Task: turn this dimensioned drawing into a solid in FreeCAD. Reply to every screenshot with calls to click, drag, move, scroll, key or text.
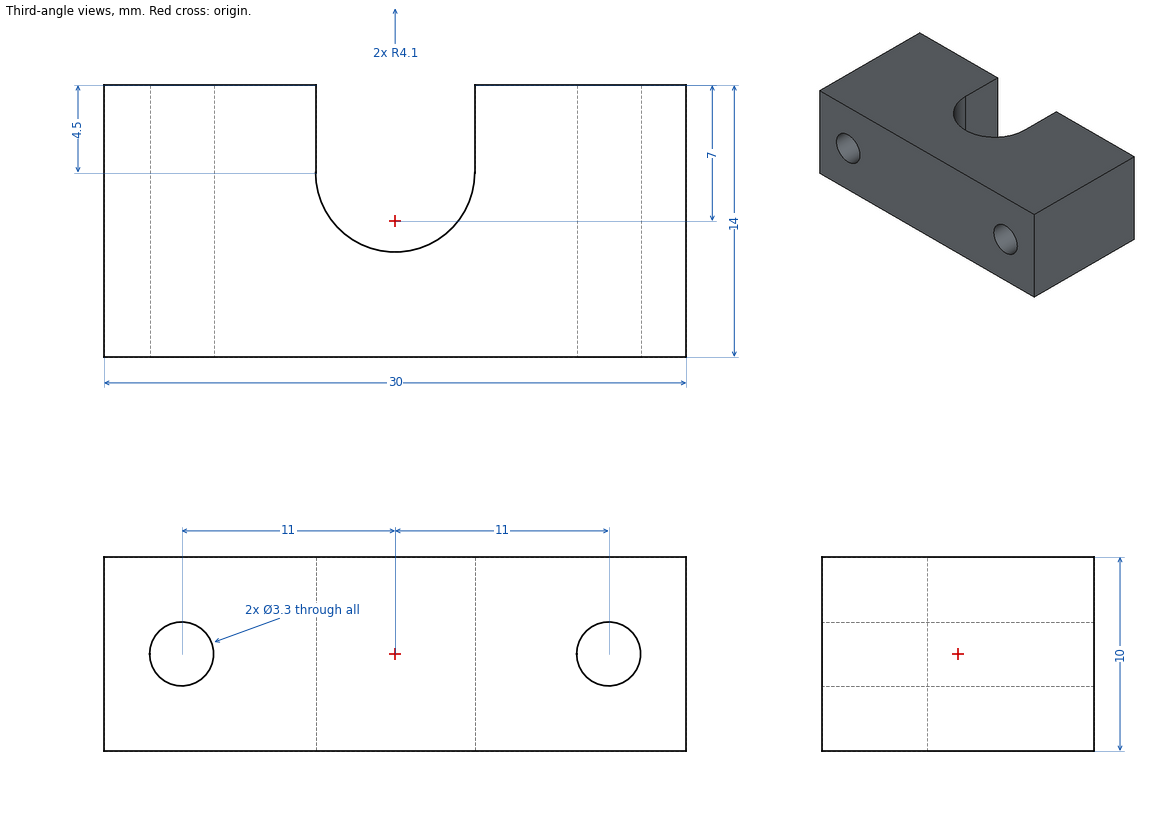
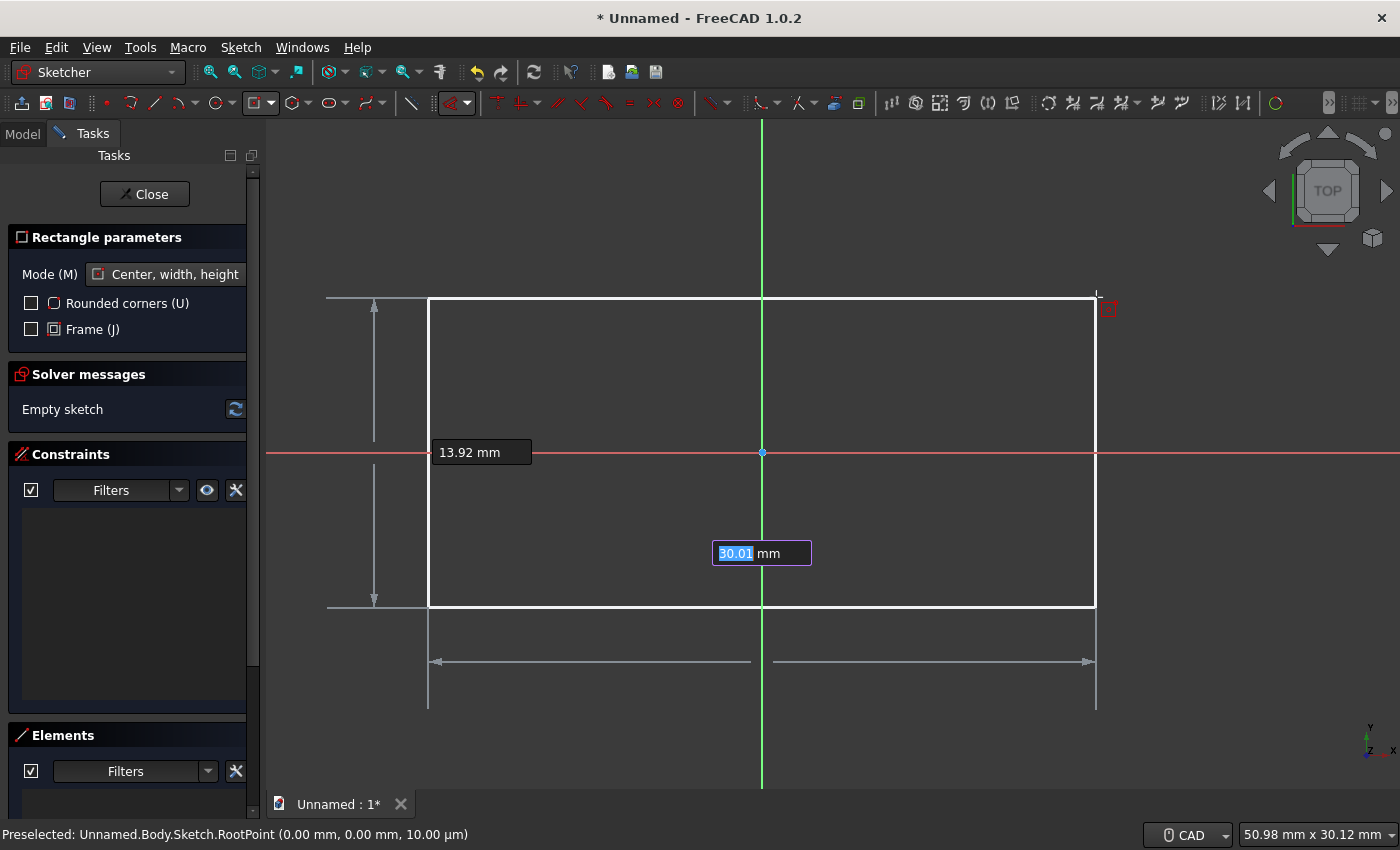
text(30)
key(Tab)
text(14)
key(Return)
key(Escape)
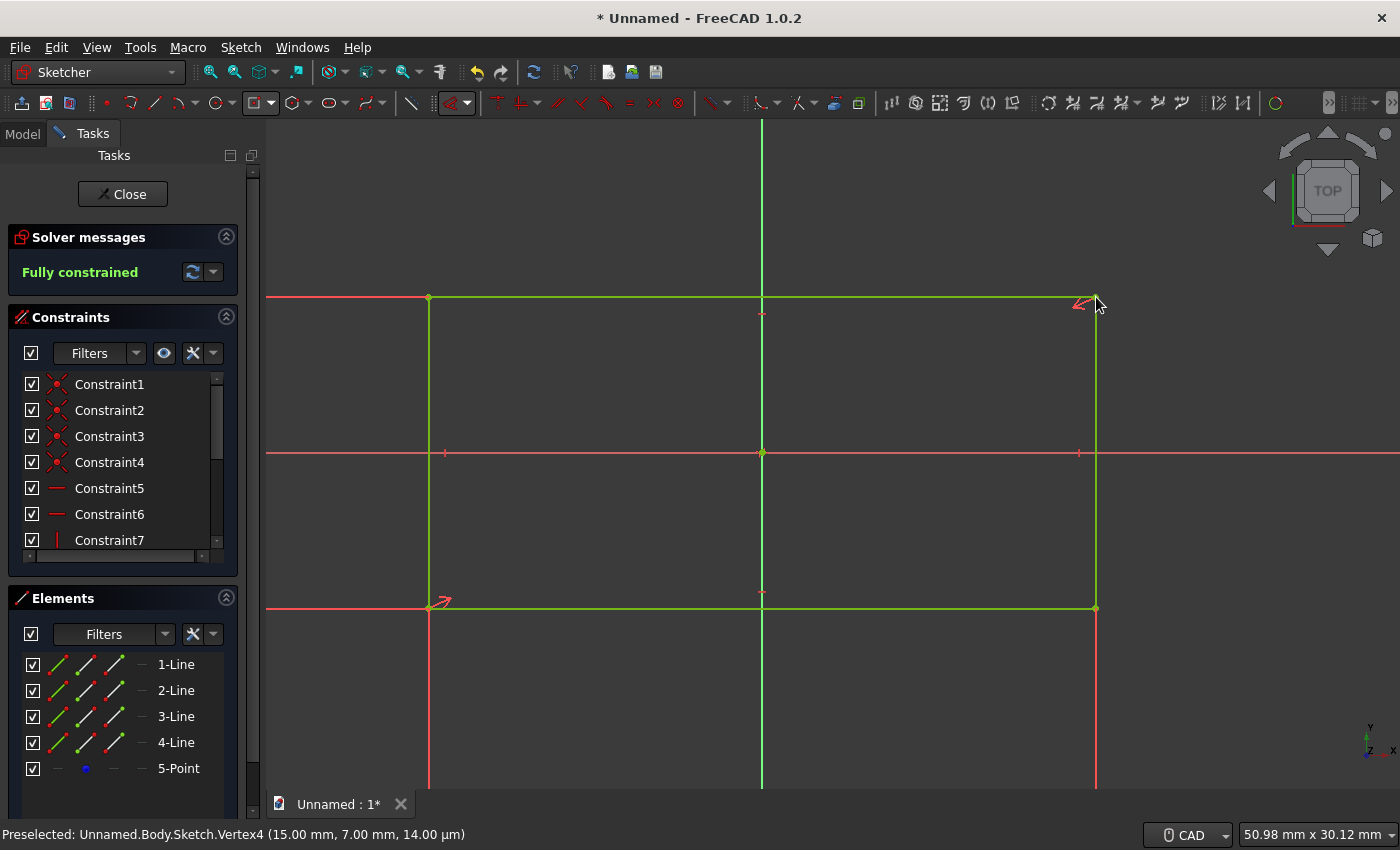
click(123, 194)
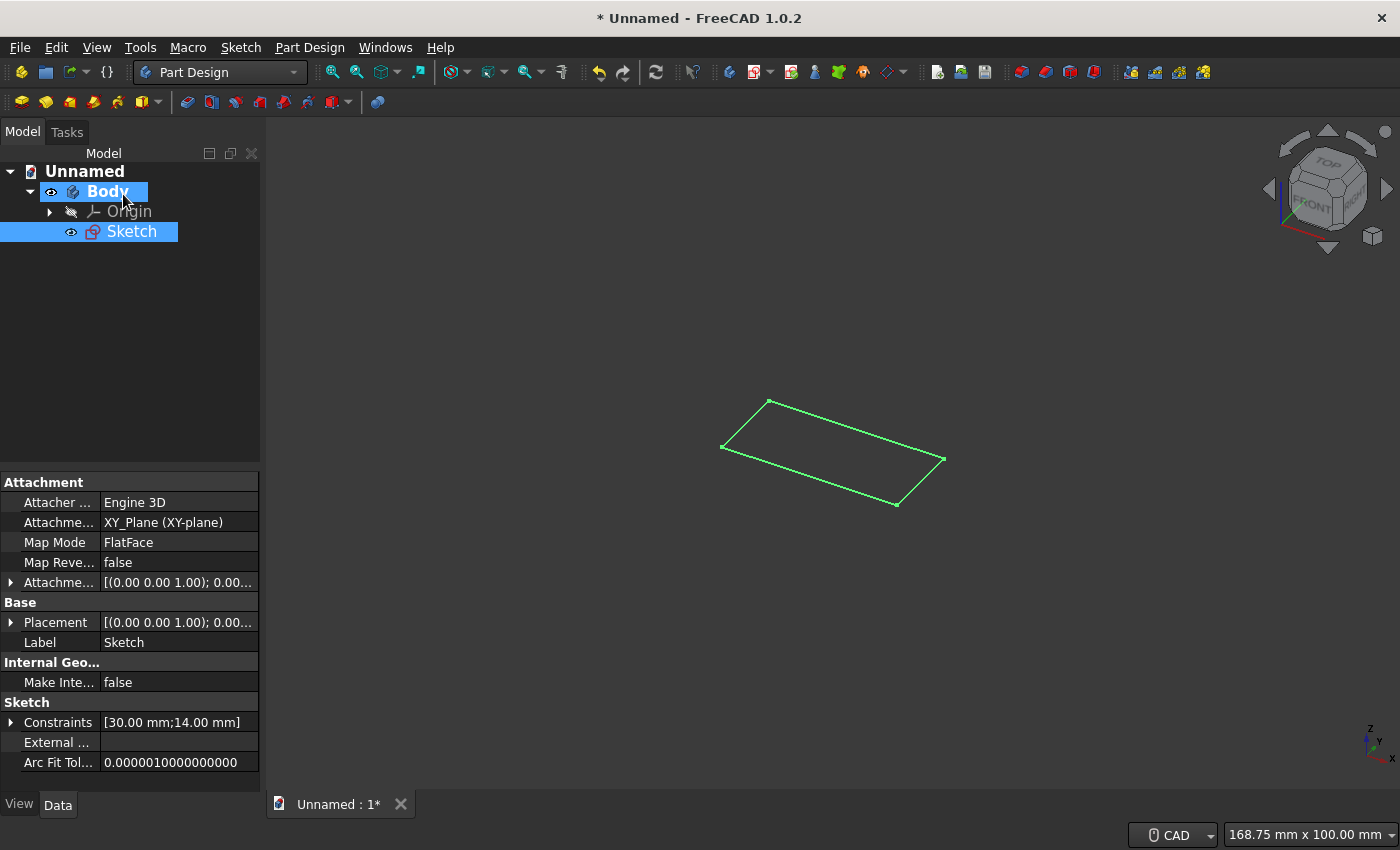
click(22, 102)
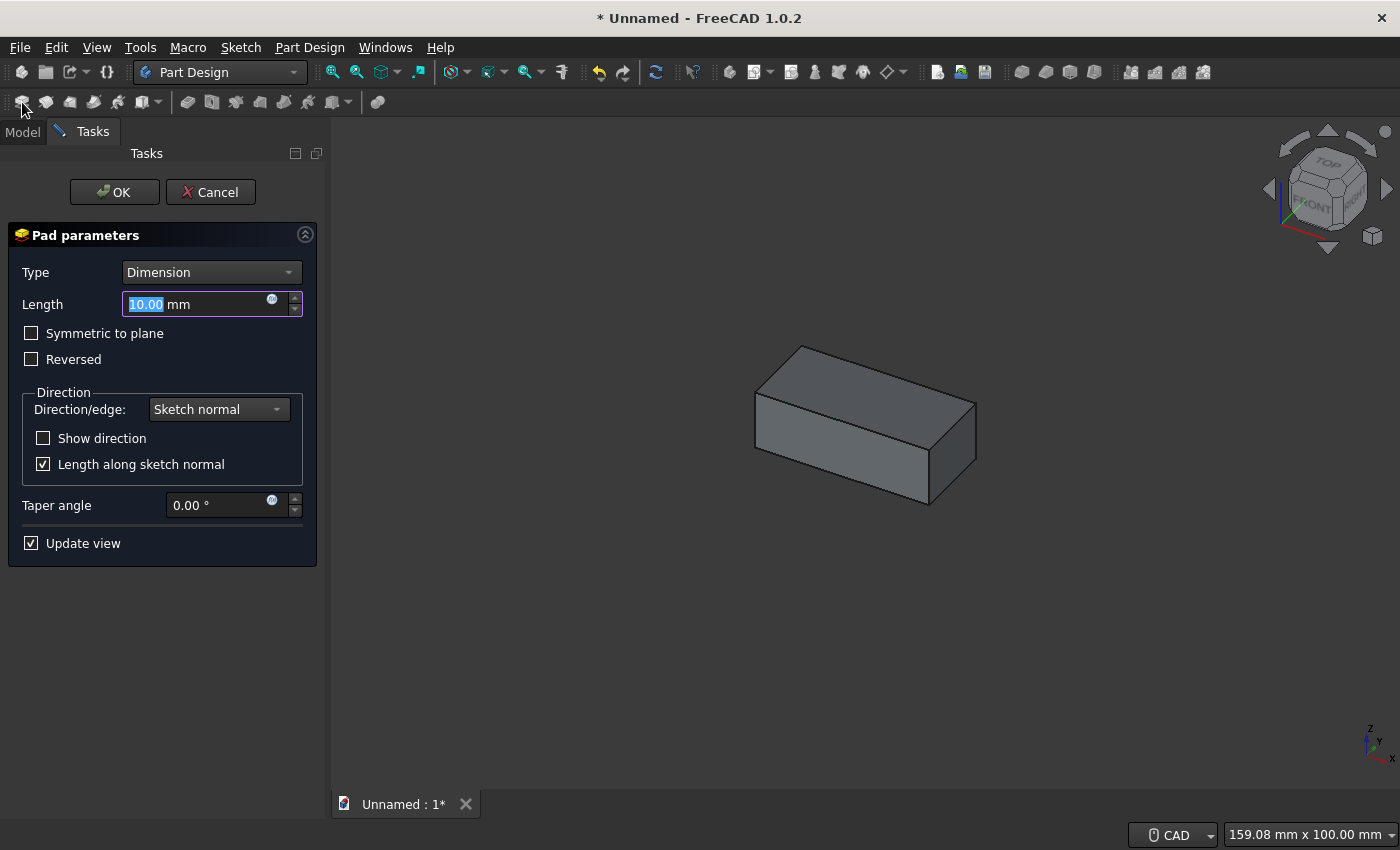
text(10)
key(Tab)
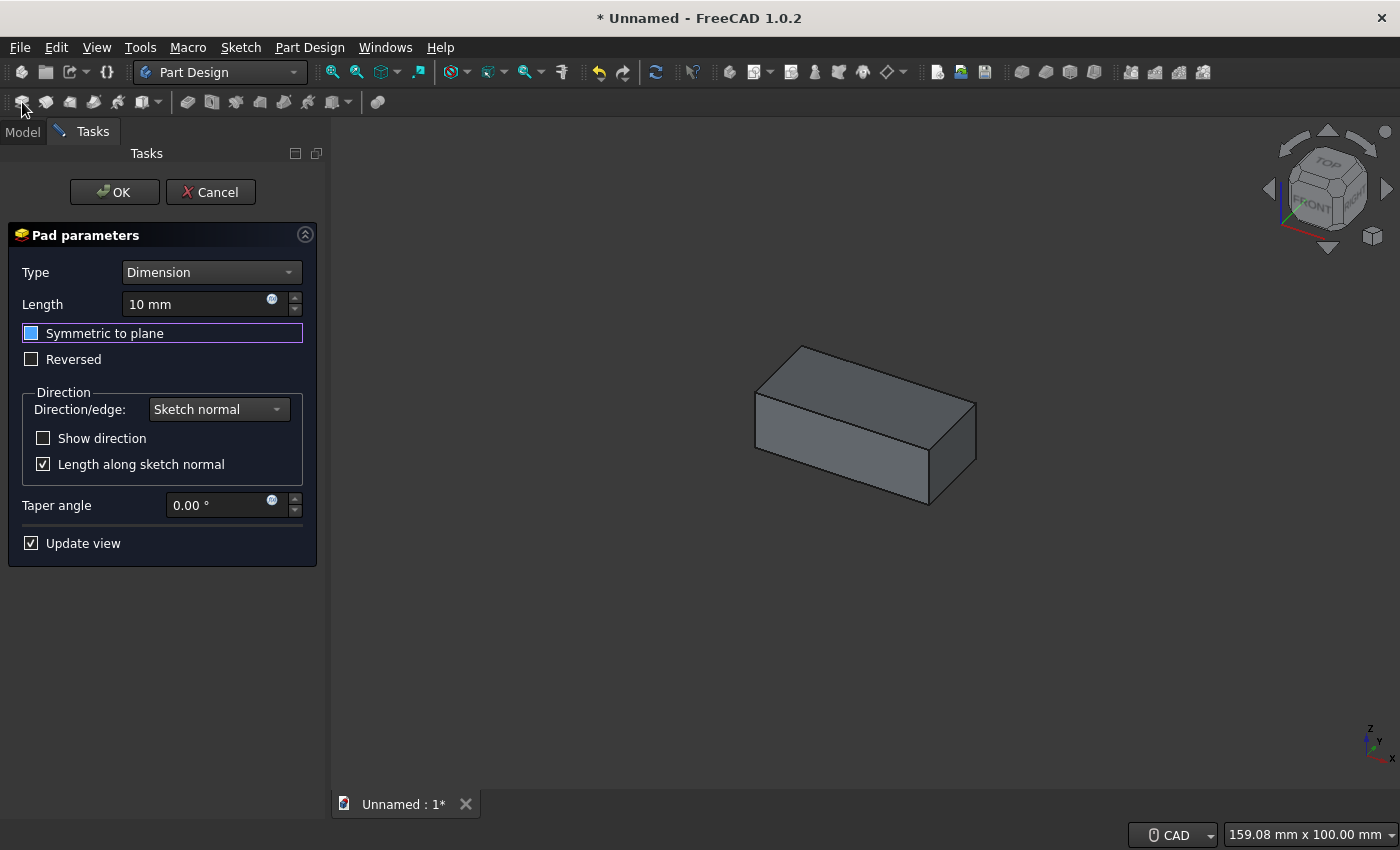
click(30, 333)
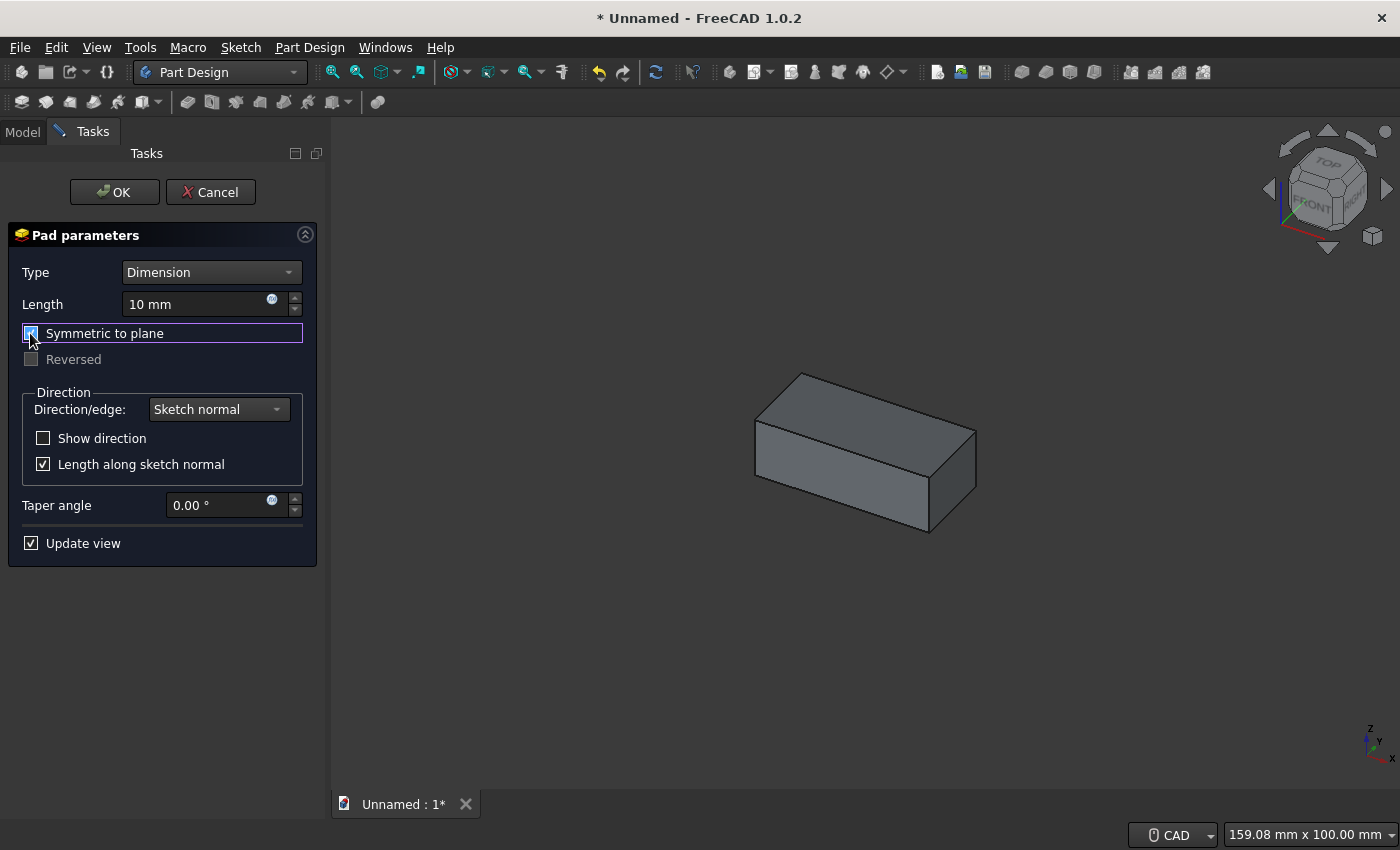
click(115, 192)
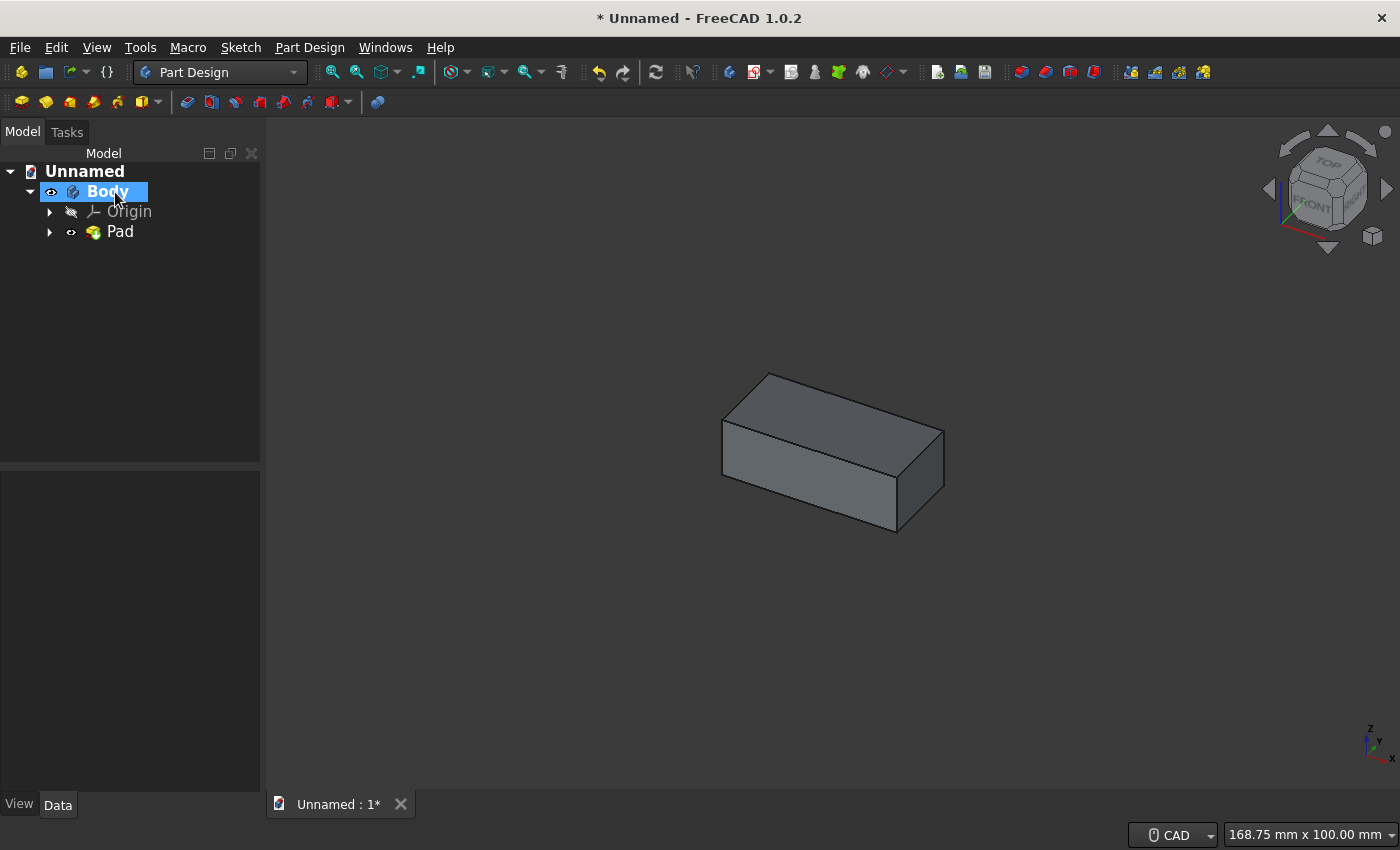
click(334, 72)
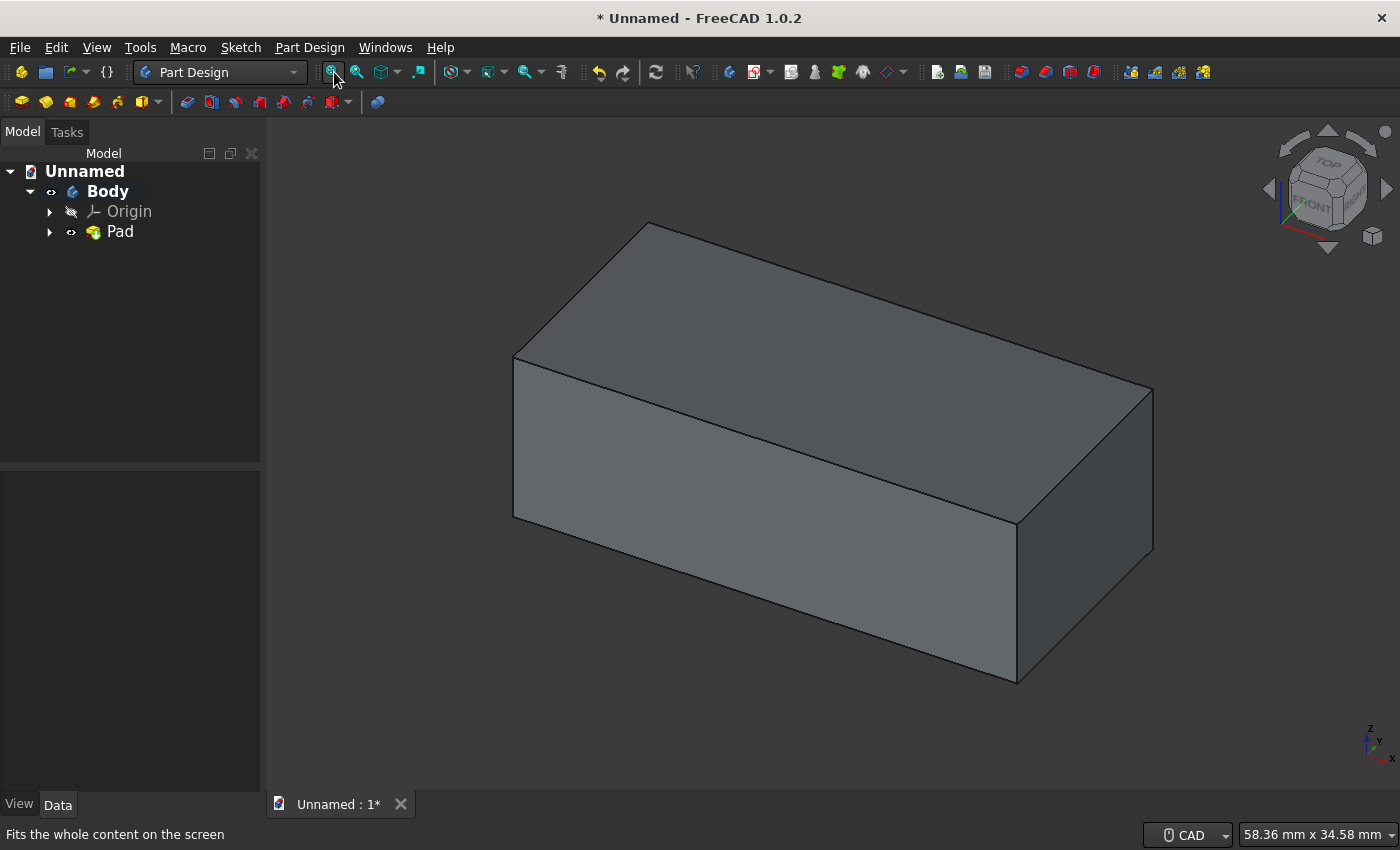
click(905, 396)